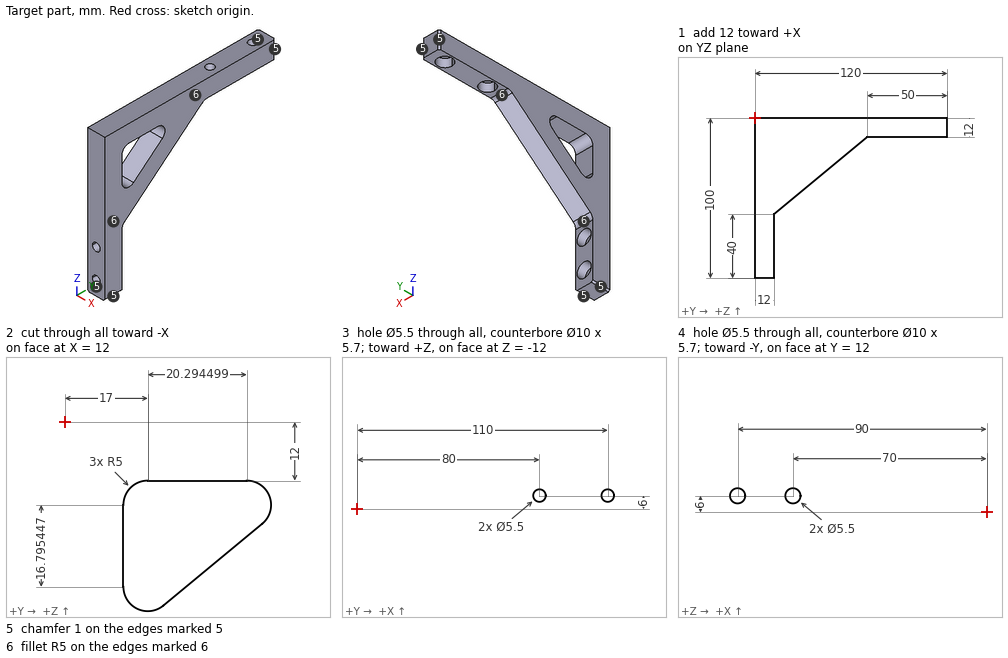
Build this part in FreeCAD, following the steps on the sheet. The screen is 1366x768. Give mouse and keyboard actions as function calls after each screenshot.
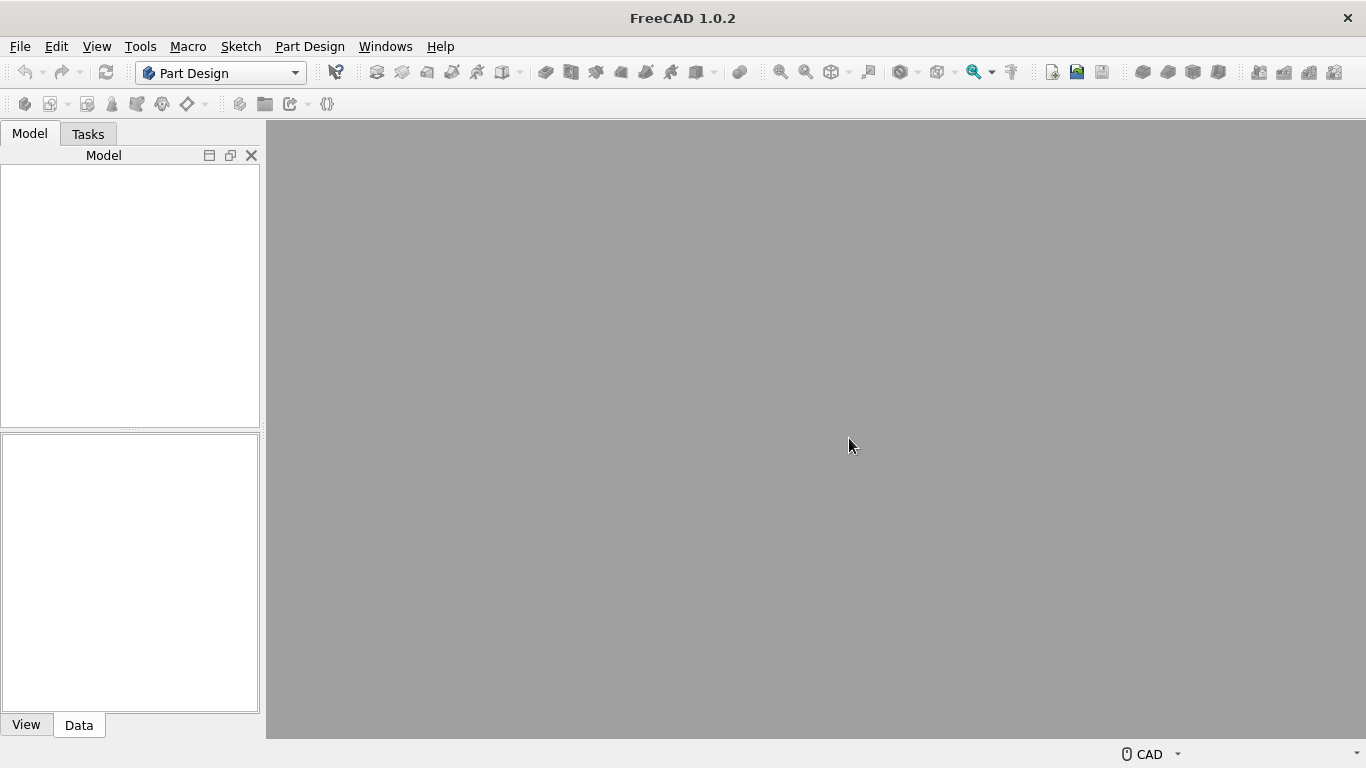
click(1052, 72)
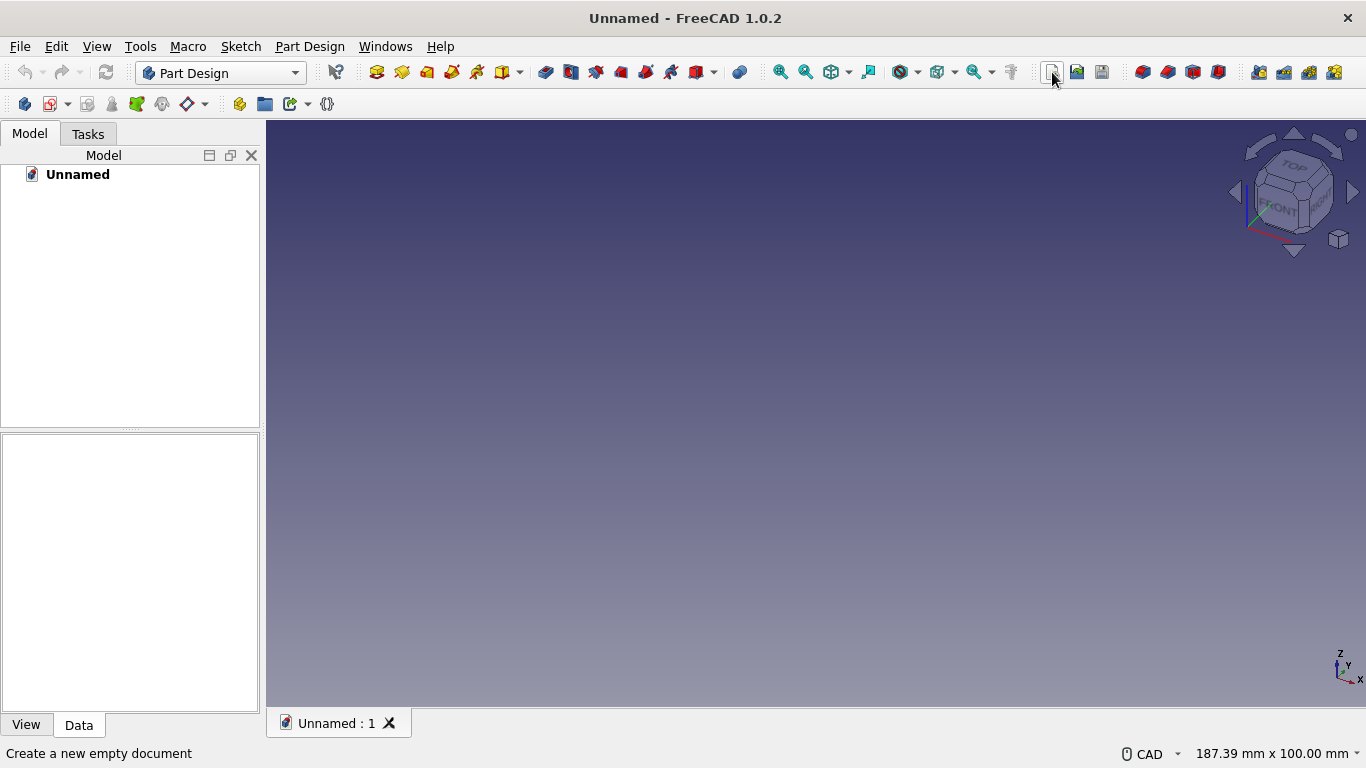
click(50, 104)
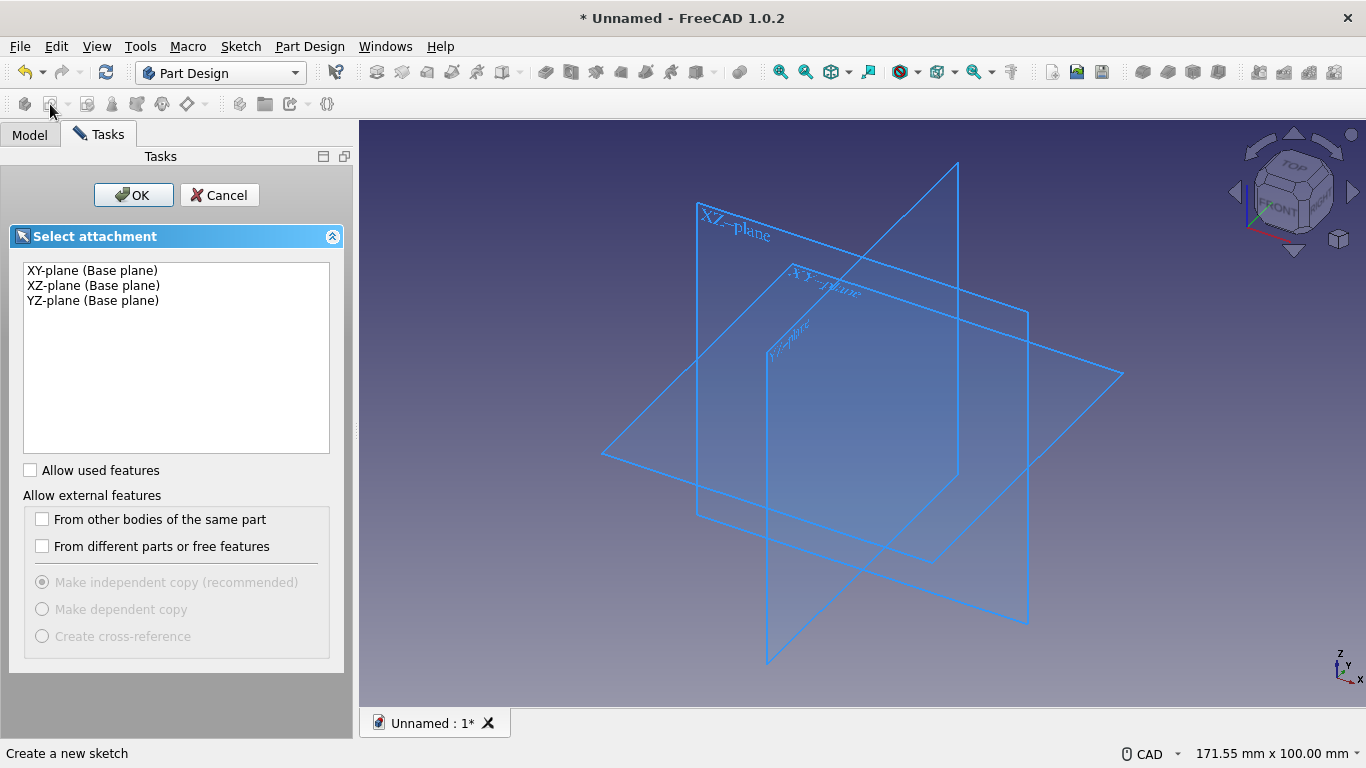
click(84, 300)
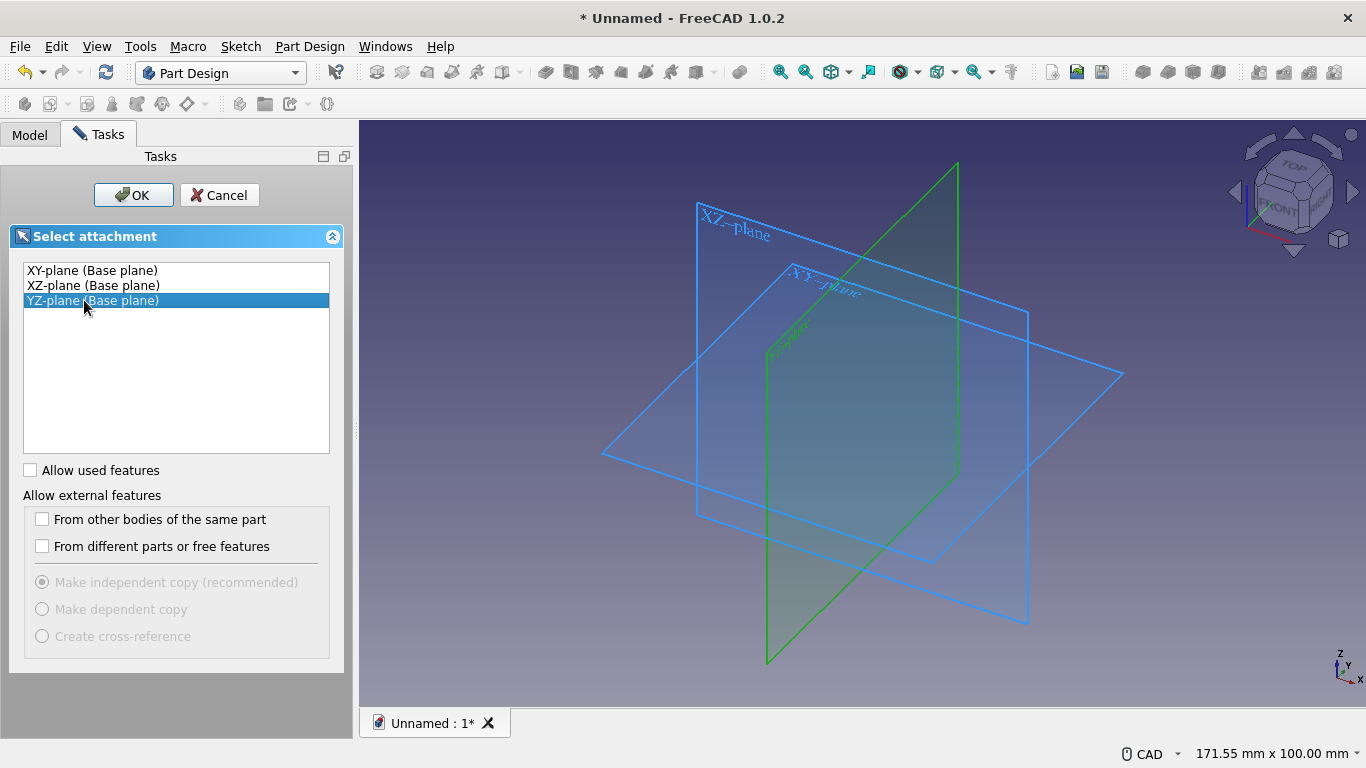
click(134, 195)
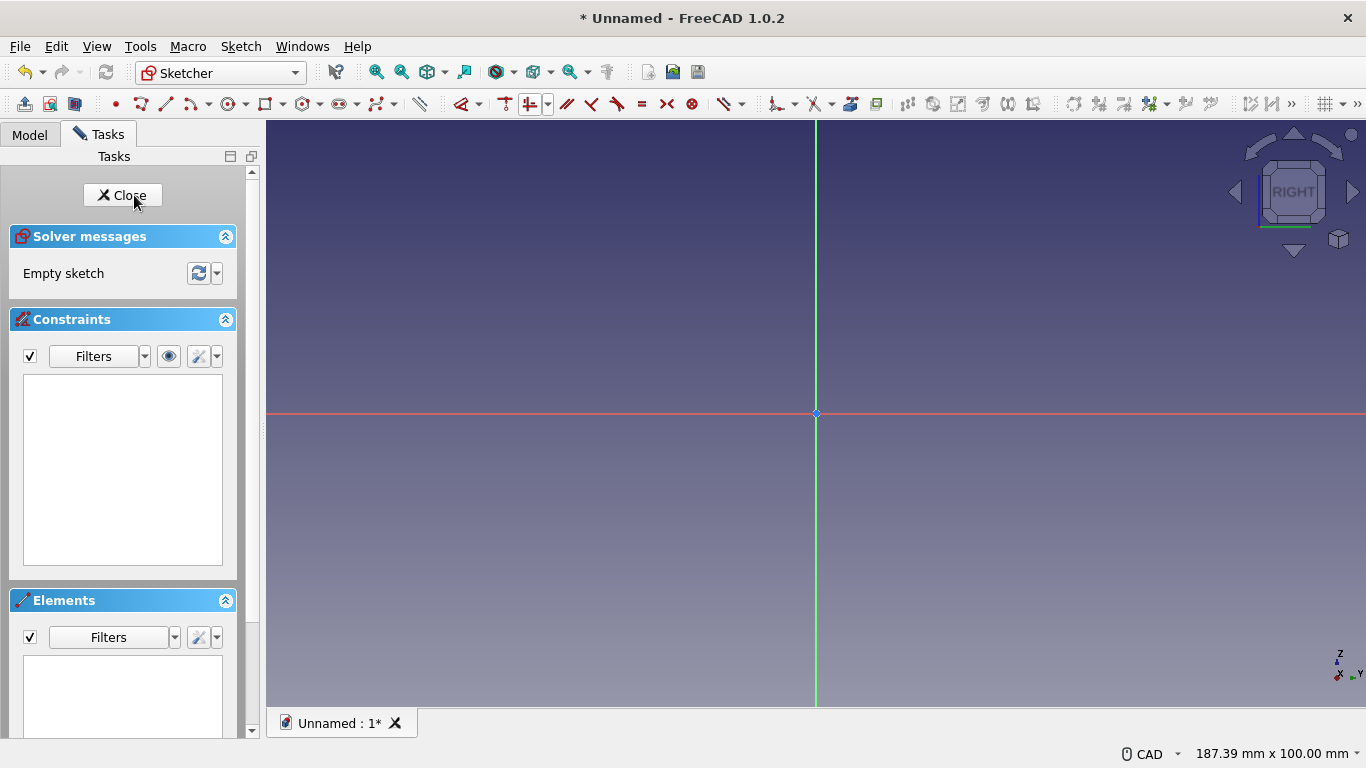
scroll(294, 148, down, 3)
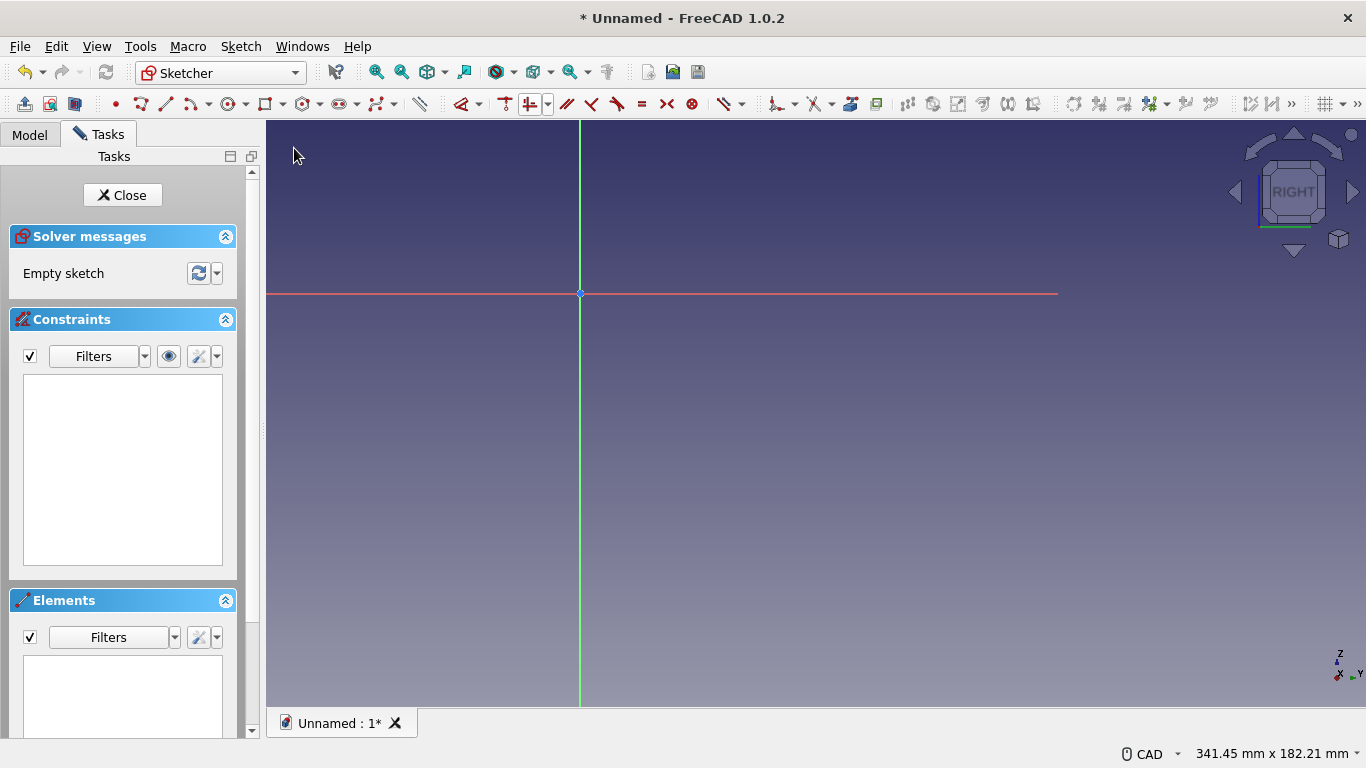
click(141, 104)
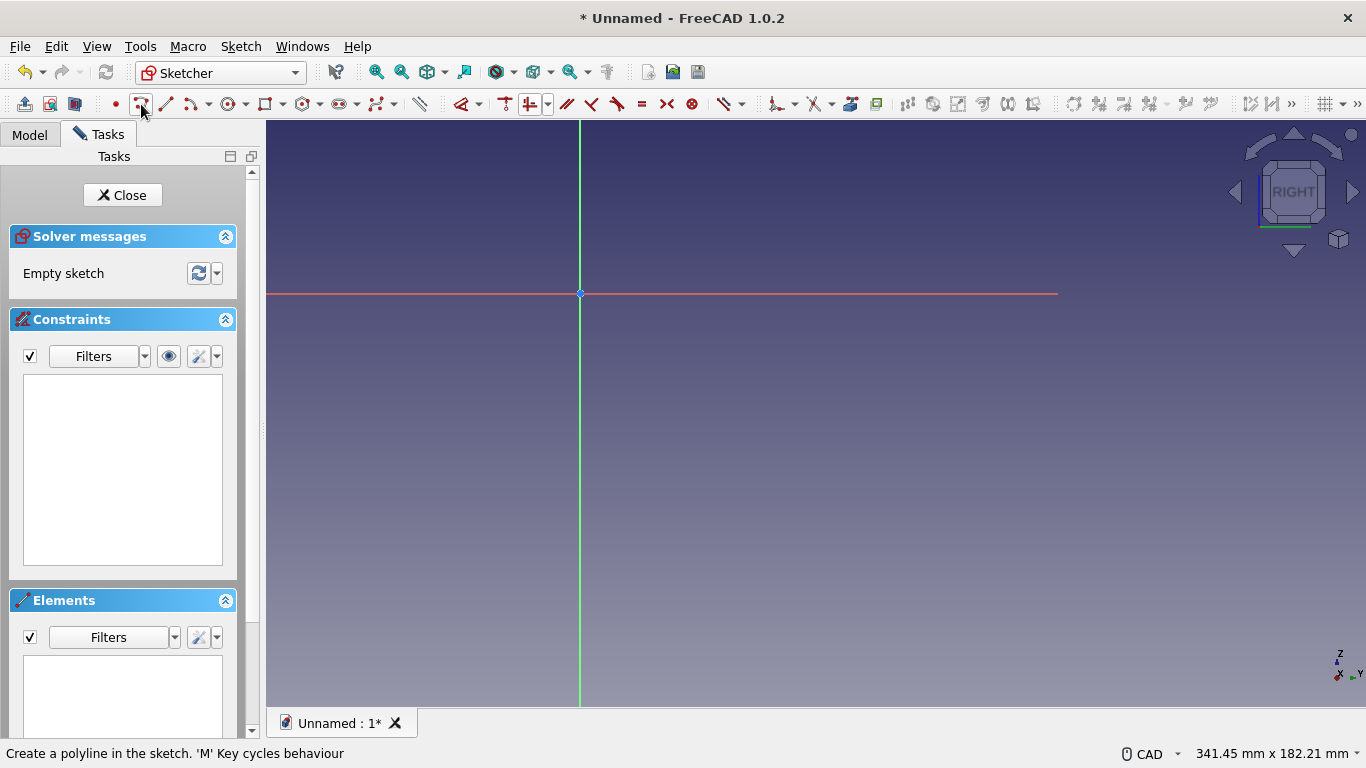
click(580, 294)
click(589, 616)
click(619, 616)
click(619, 487)
click(806, 332)
click(967, 332)
click(967, 303)
click(580, 294)
key(Escape)
key(Escape)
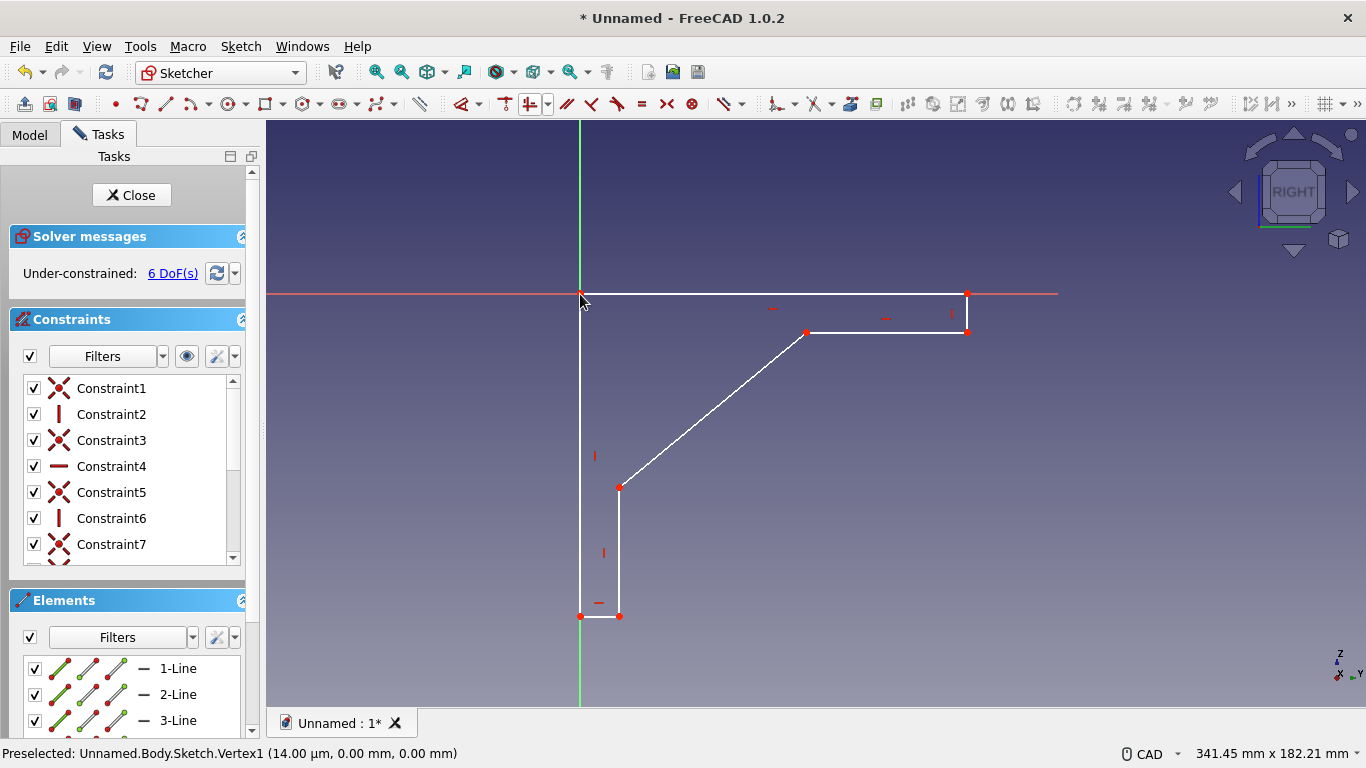
click(460, 104)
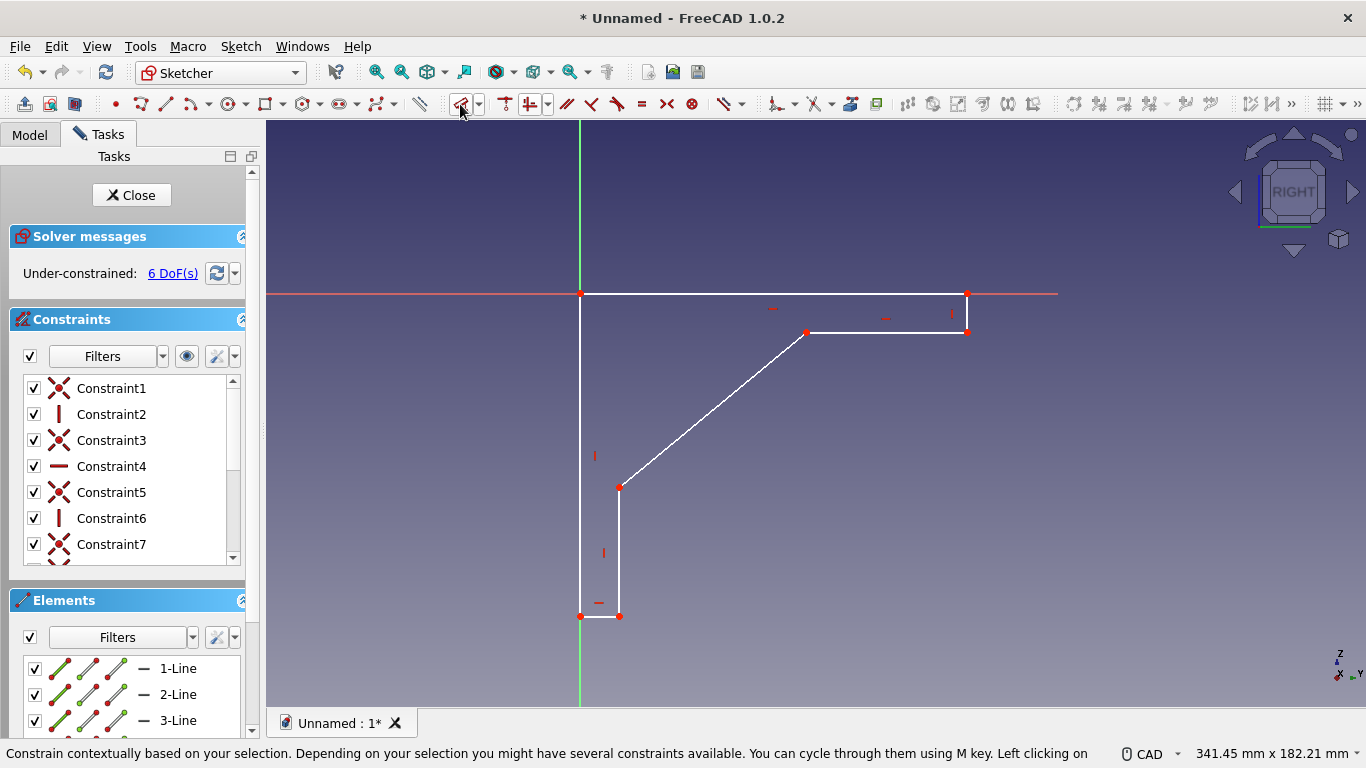
click(592, 617)
click(600, 651)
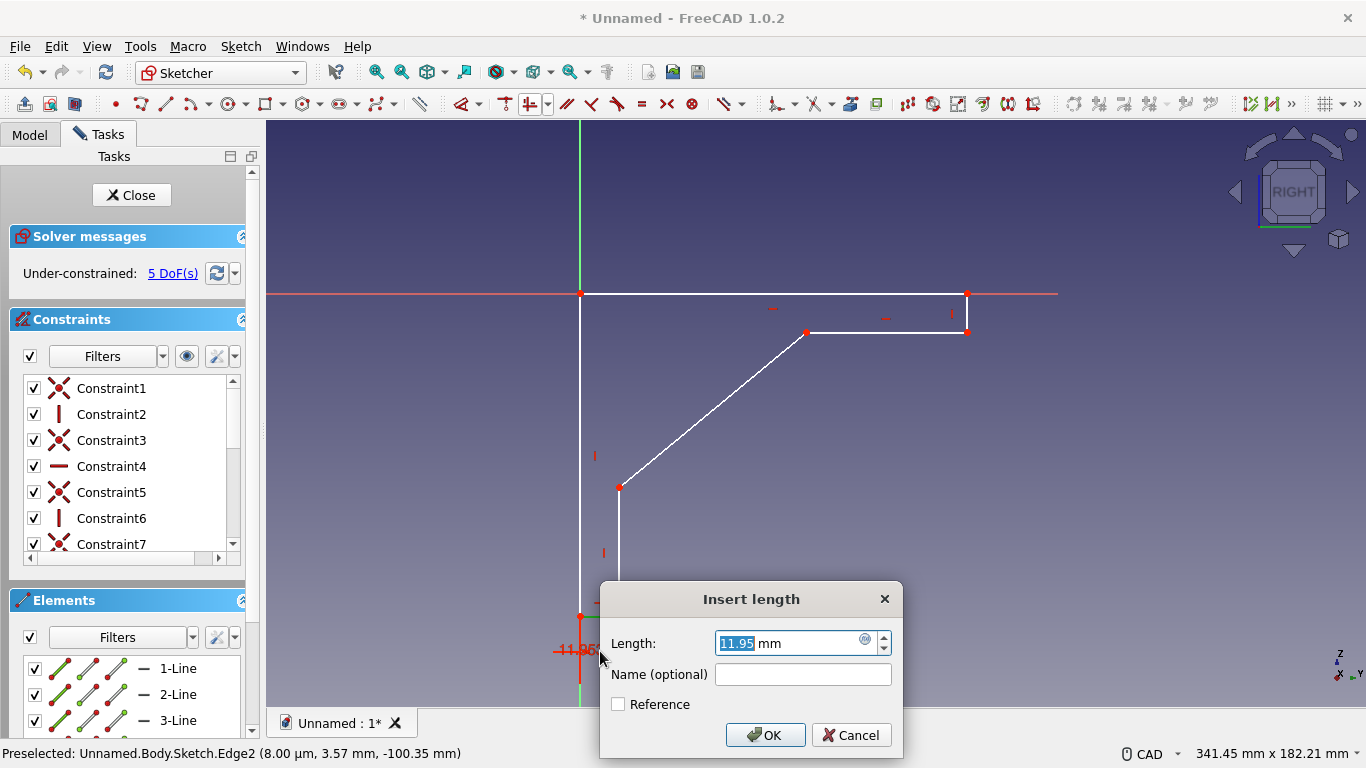
text(12)
key(Return)